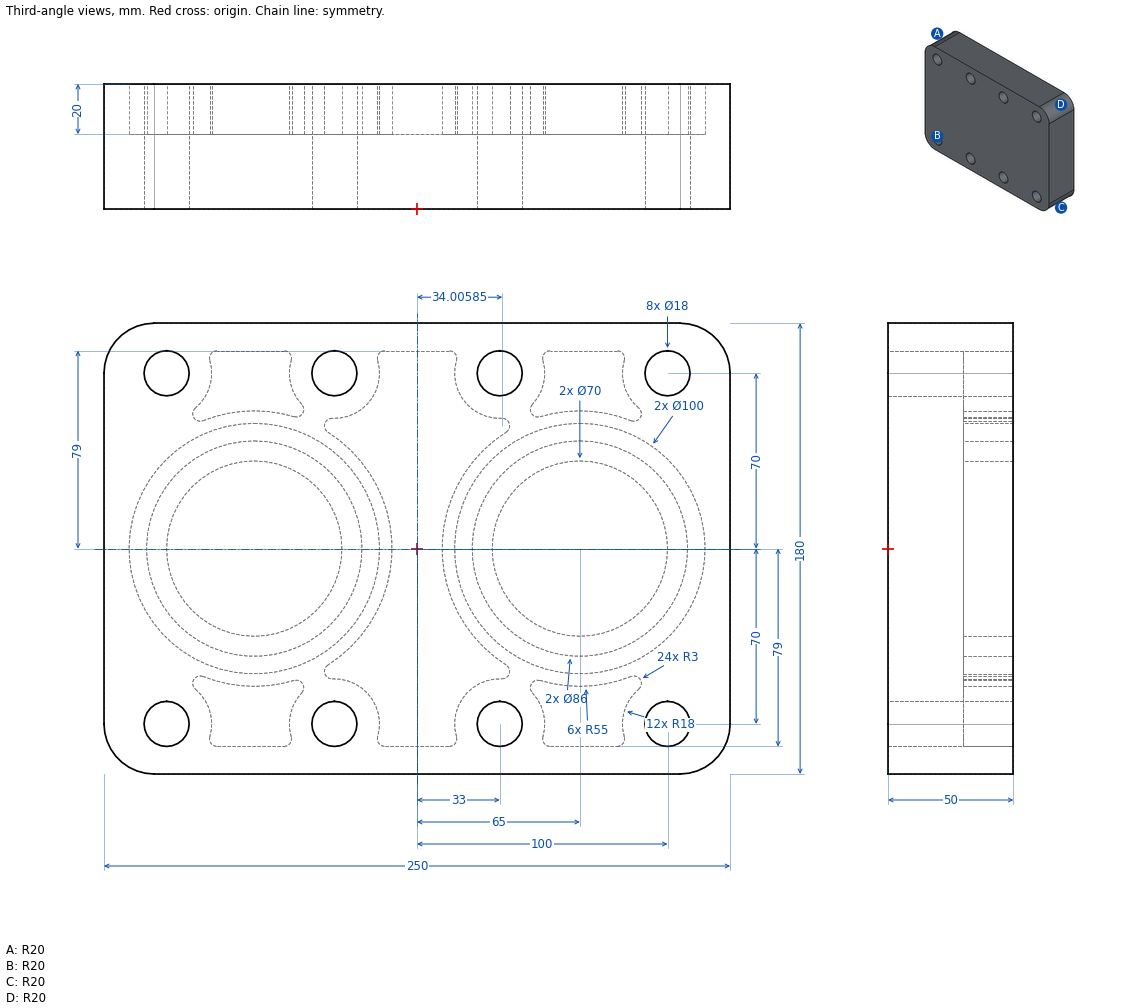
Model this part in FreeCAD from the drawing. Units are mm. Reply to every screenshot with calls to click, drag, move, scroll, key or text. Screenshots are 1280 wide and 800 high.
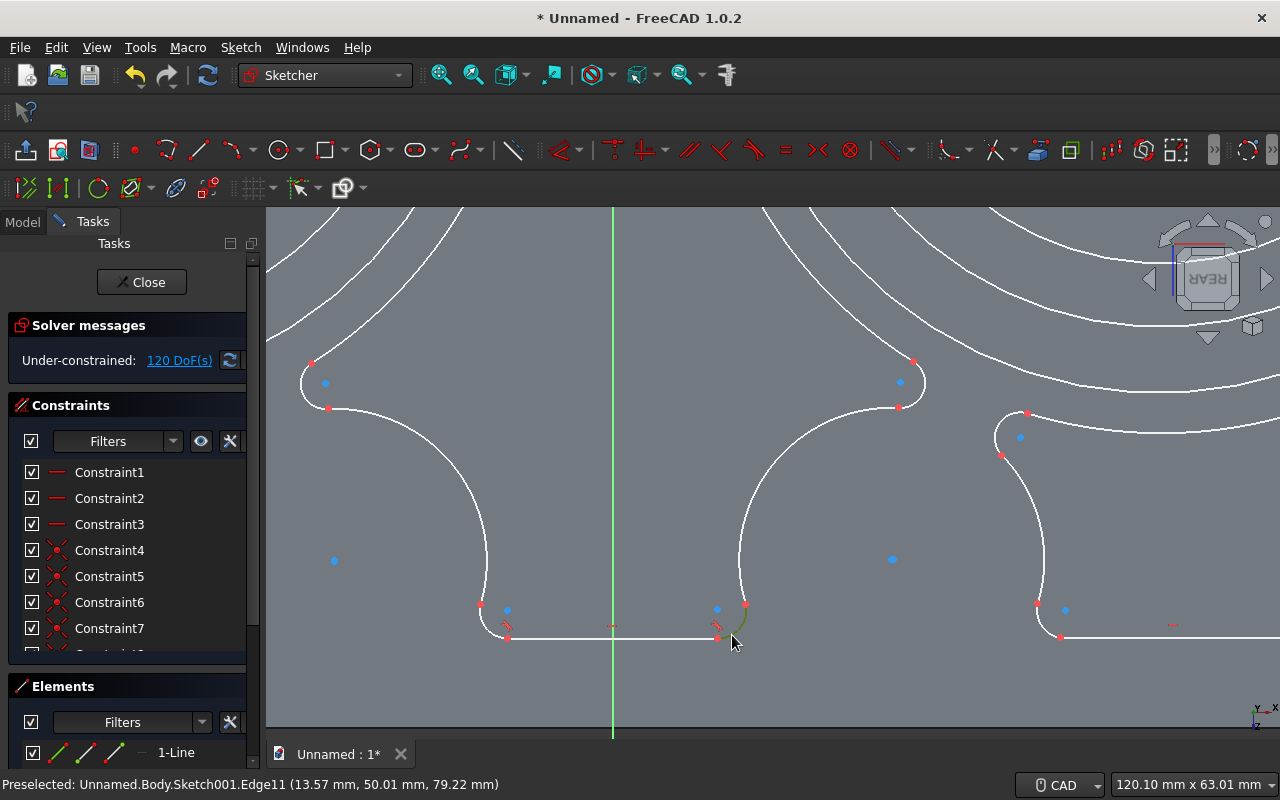
scroll(734, 638, down, 7)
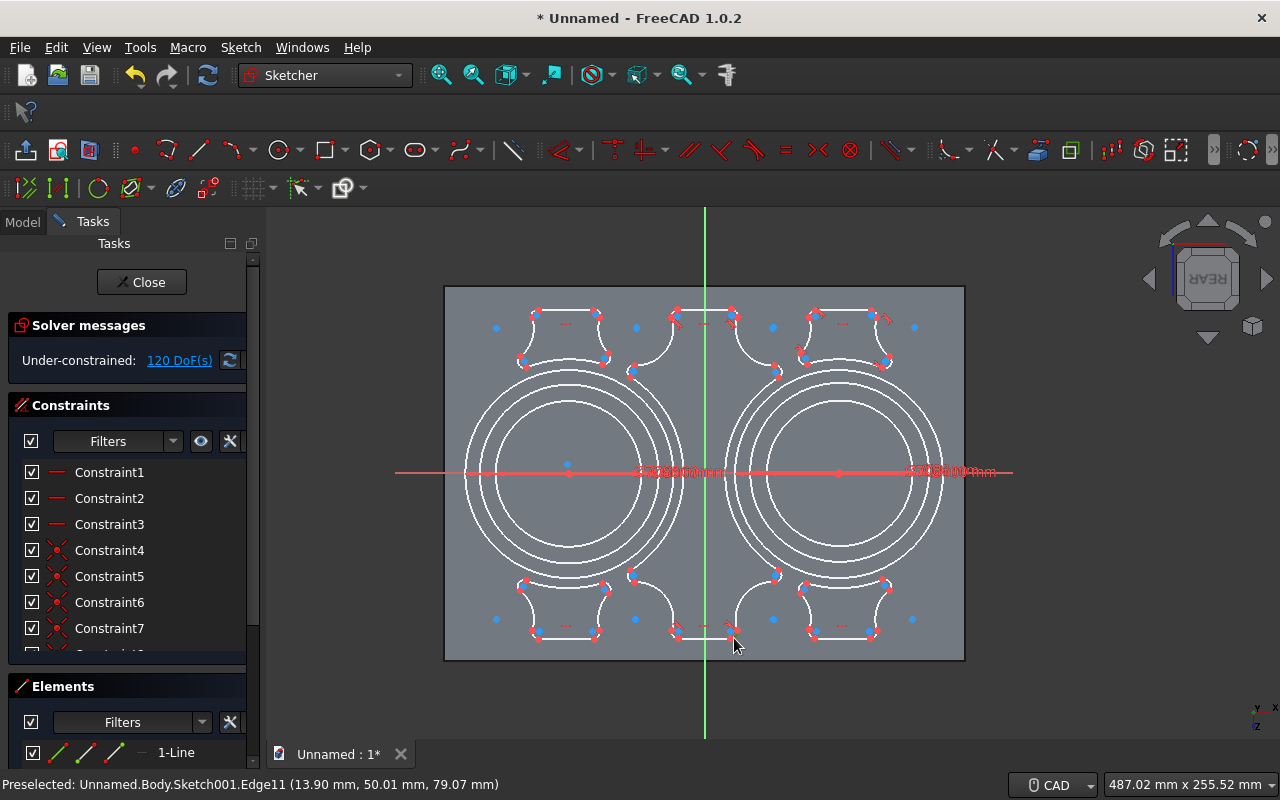
click(754, 587)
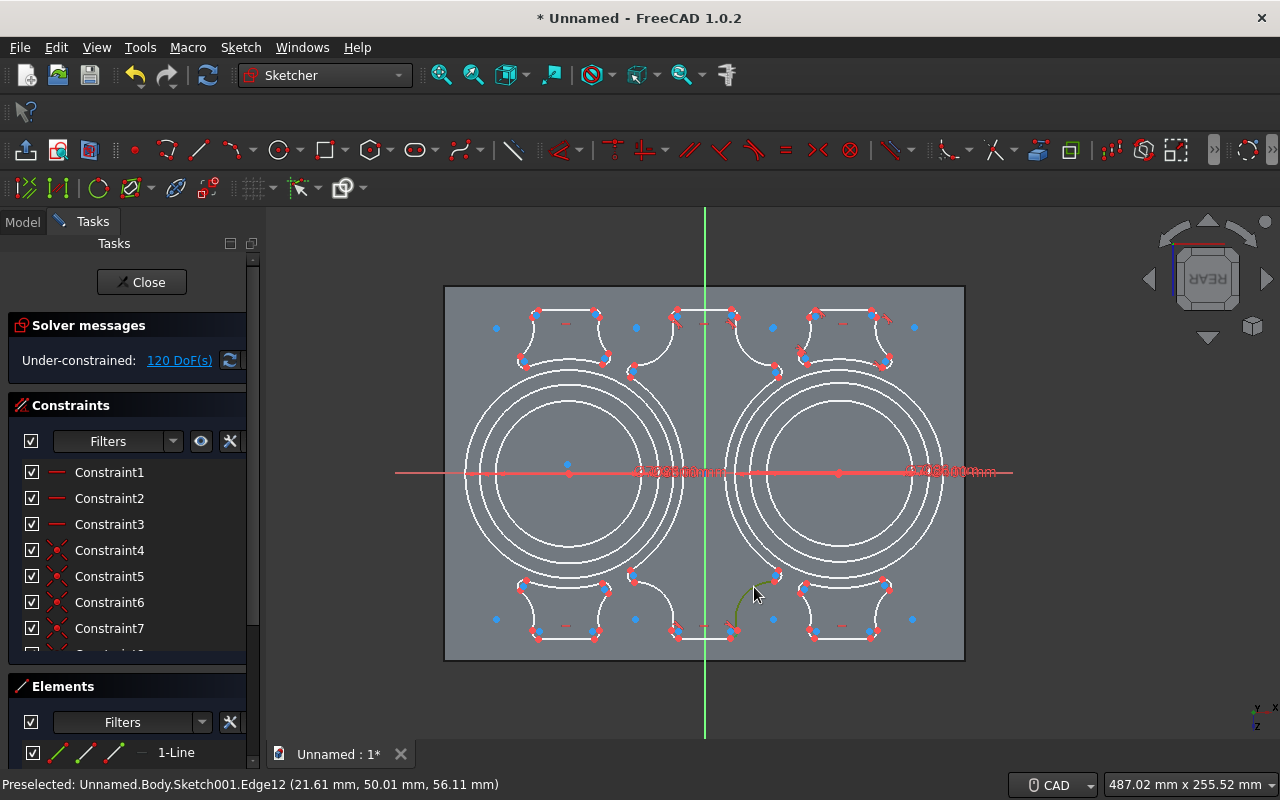
click(754, 150)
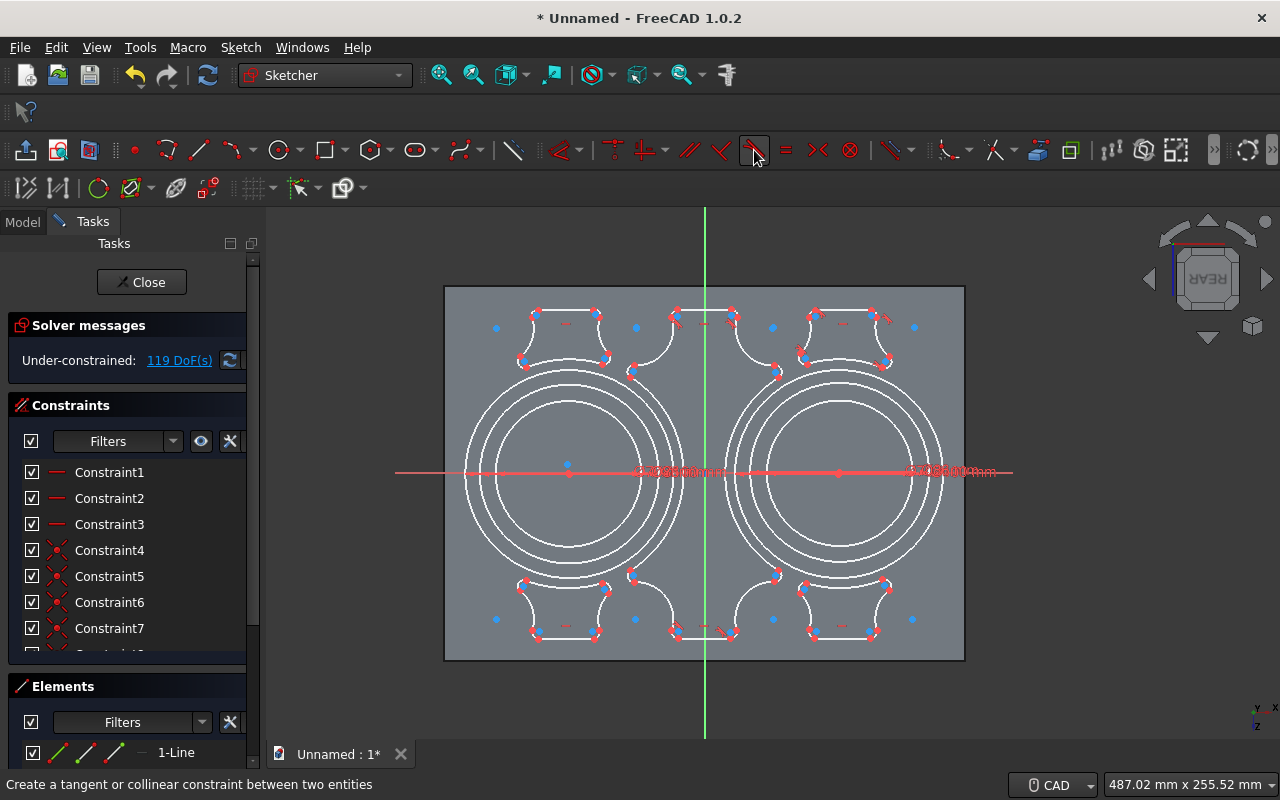
click(754, 587)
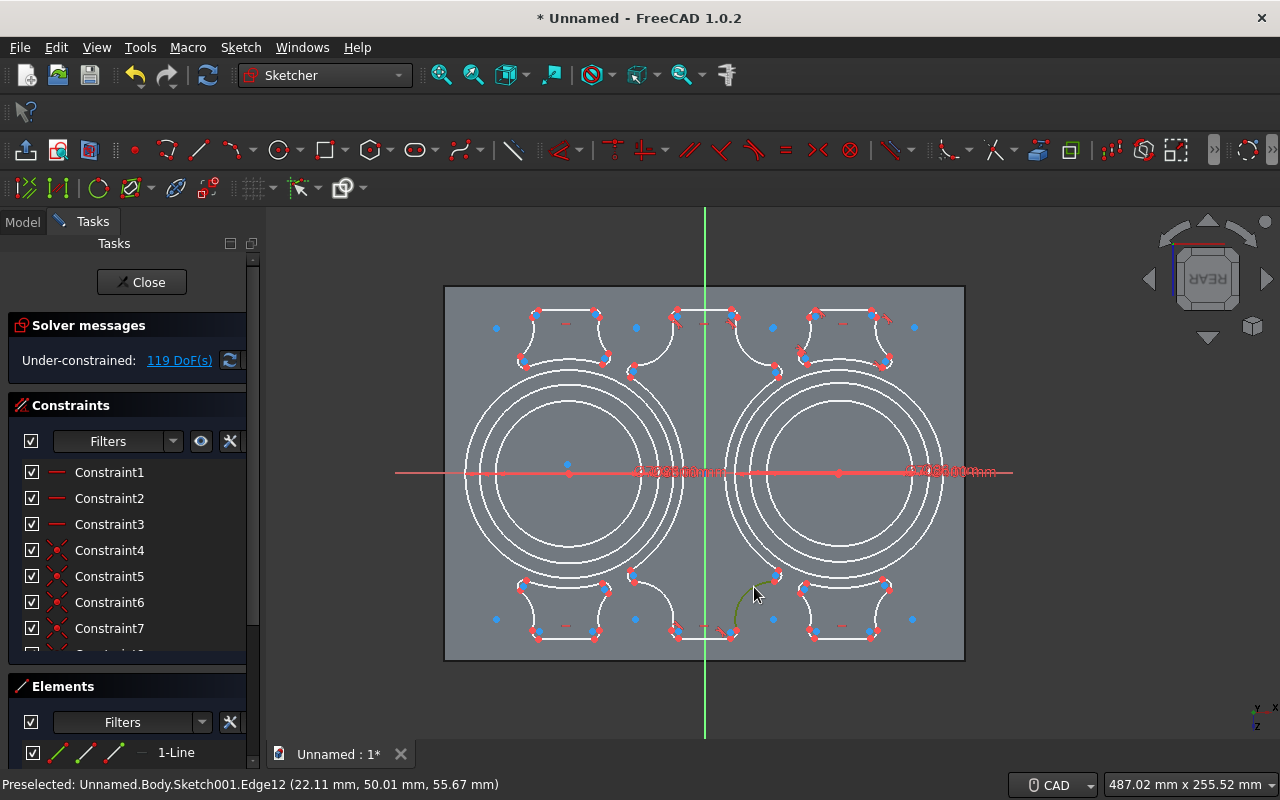
scroll(781, 578, up, 5)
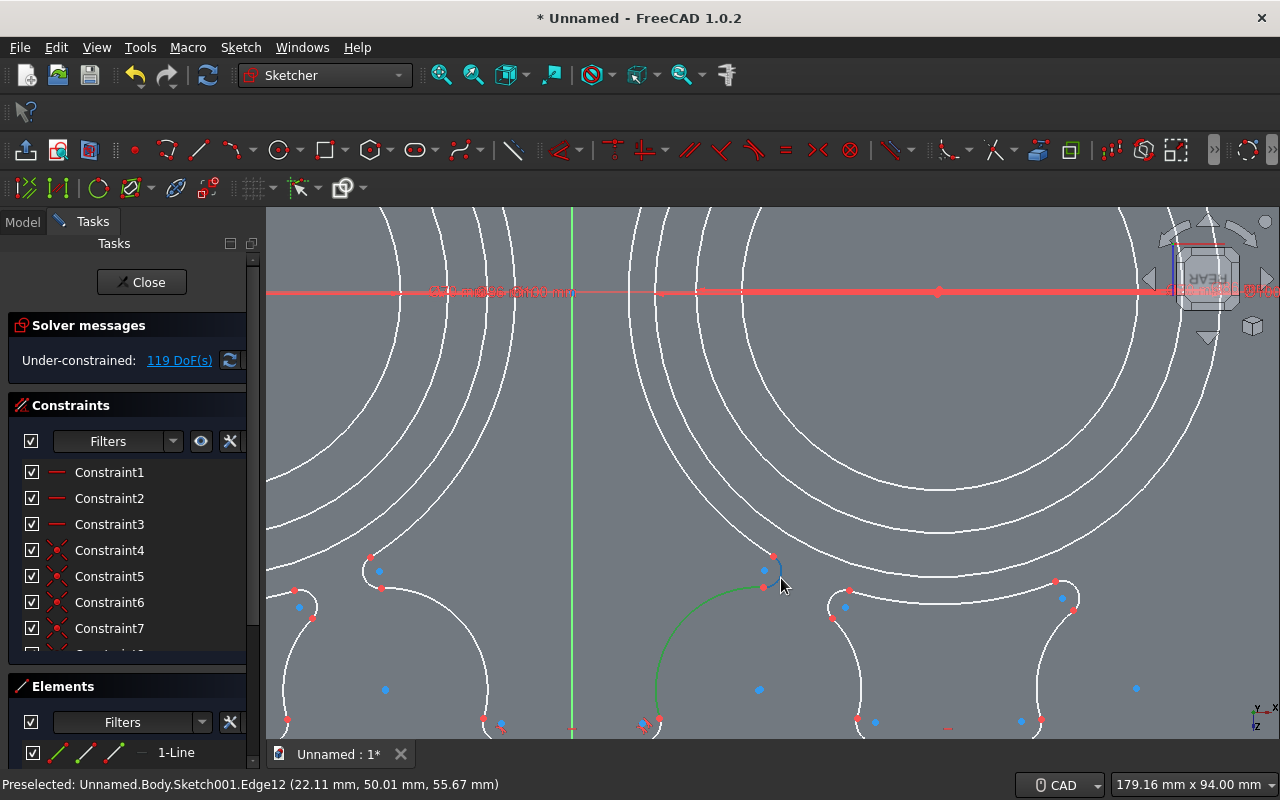
click(781, 576)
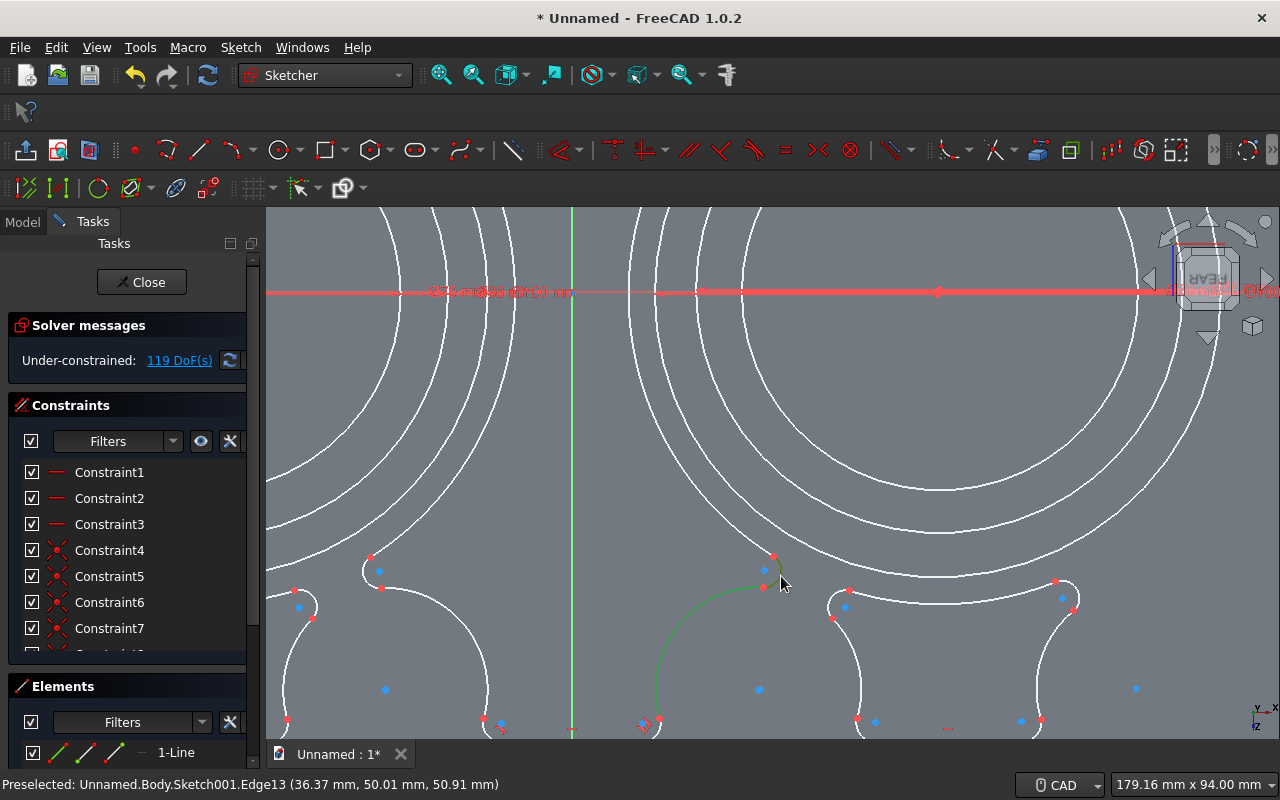
click(754, 150)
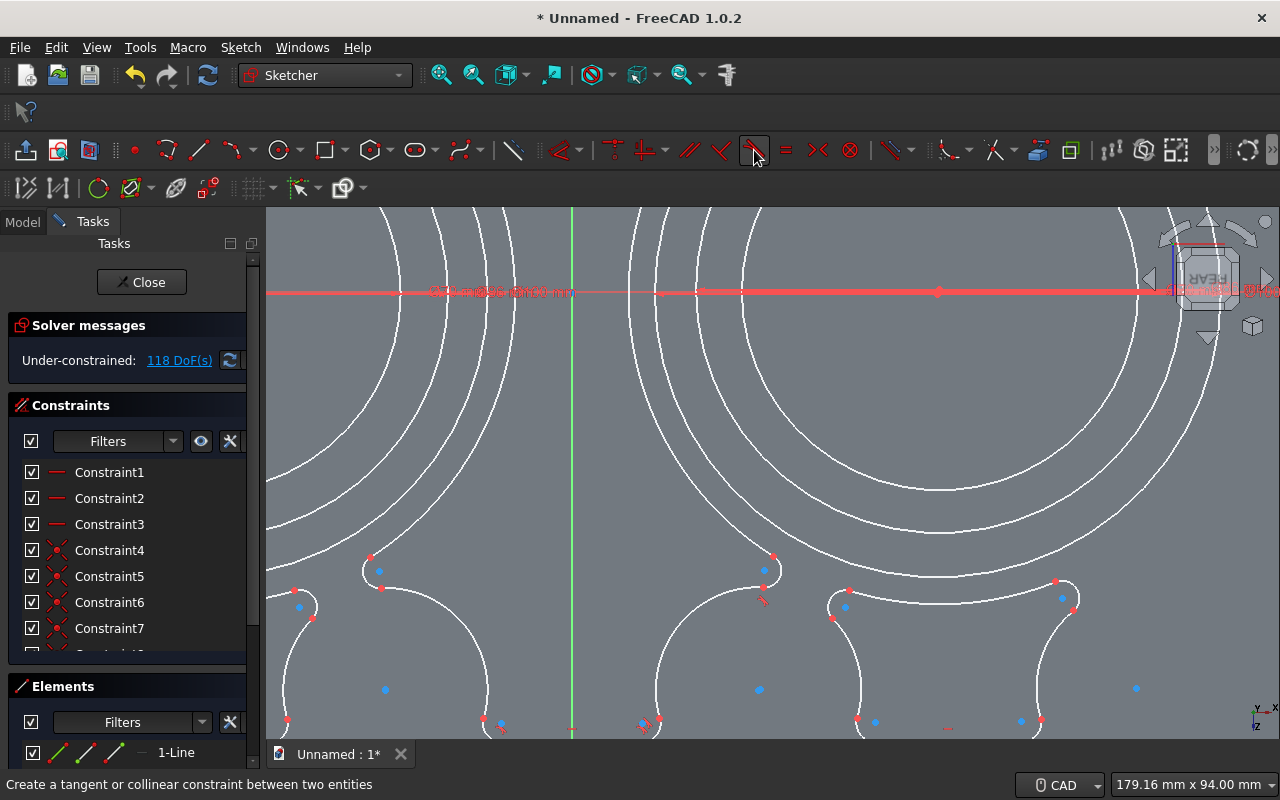
click(776, 583)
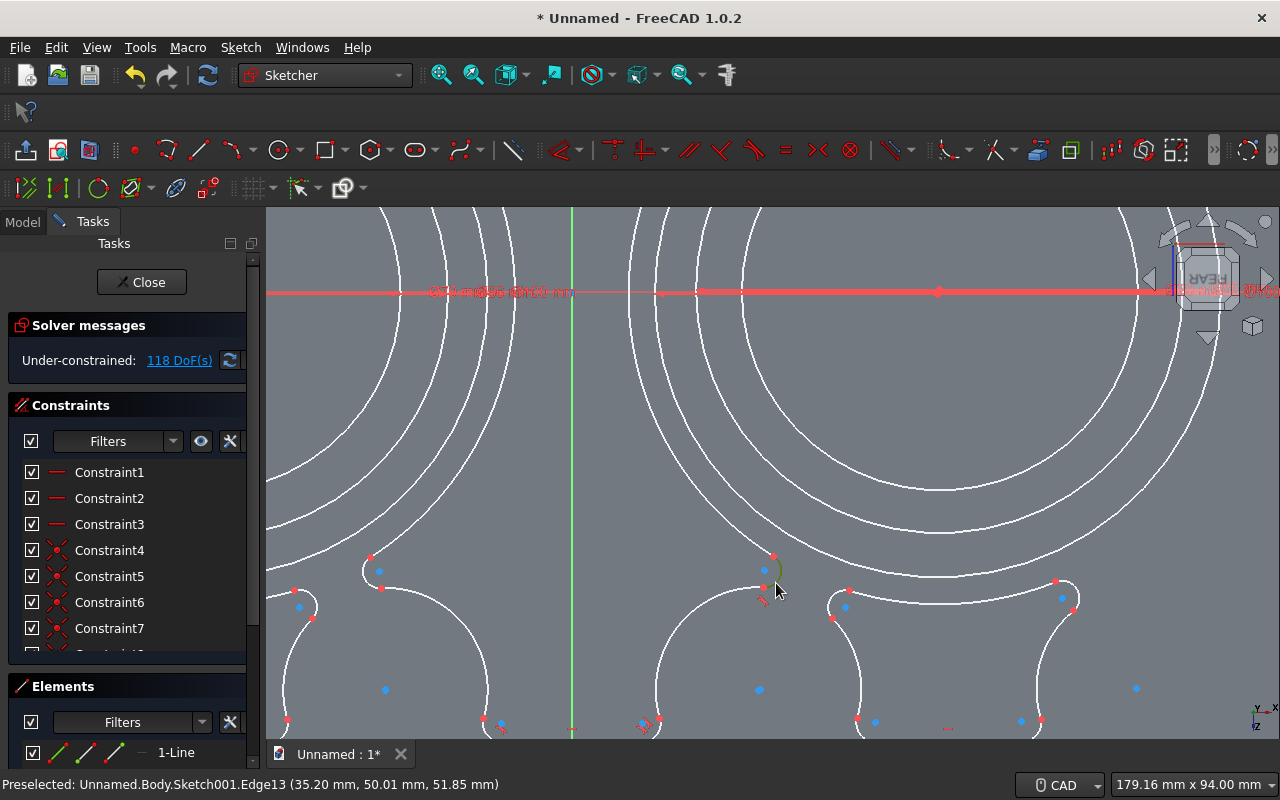
click(654, 416)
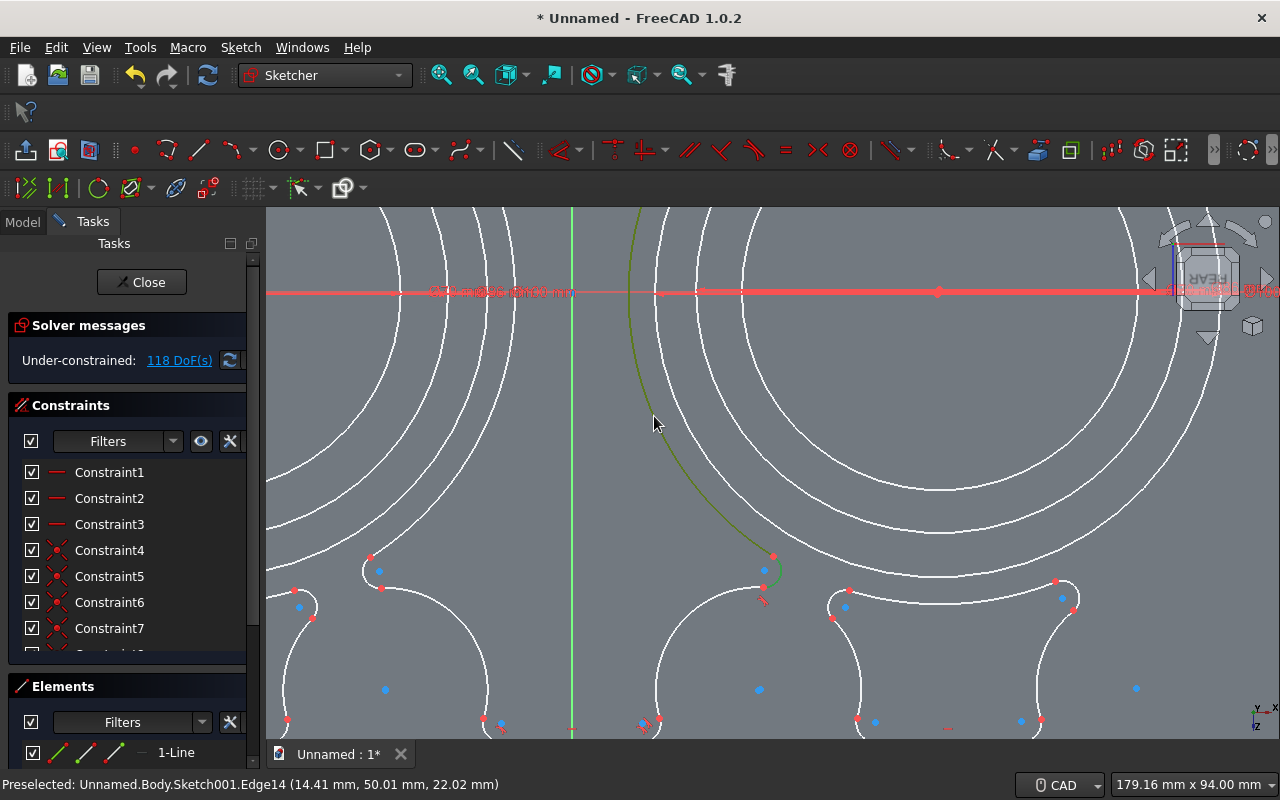
click(754, 150)